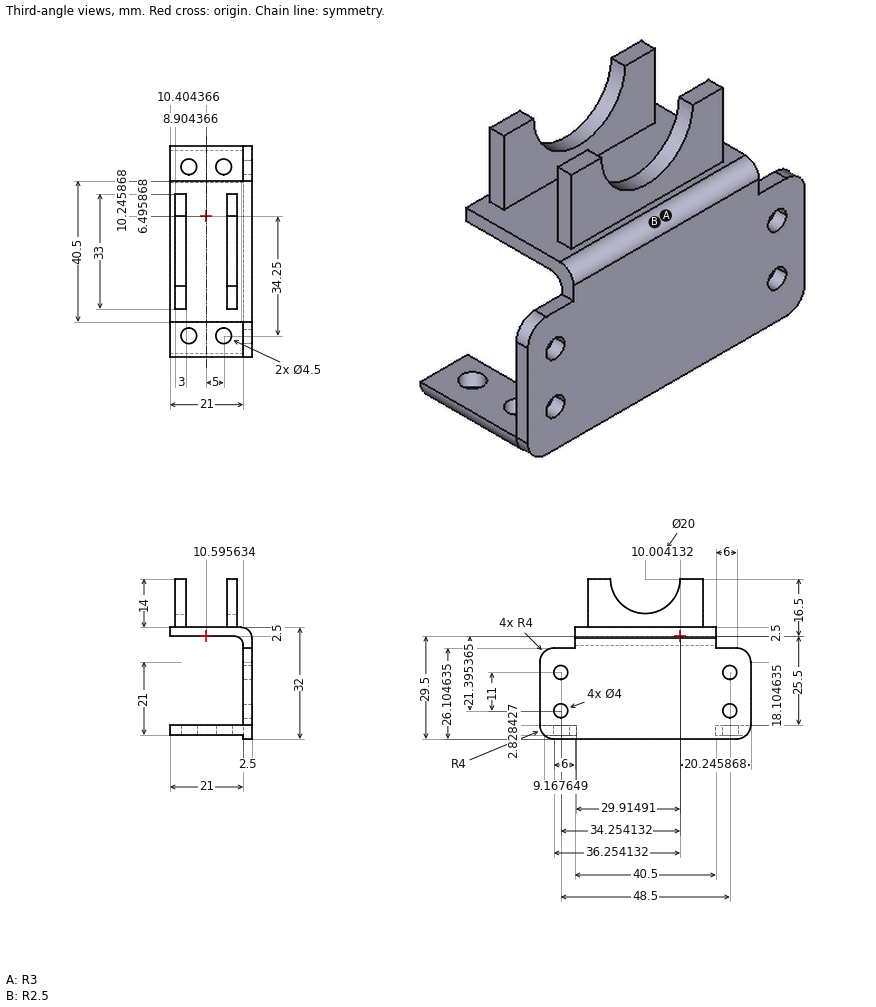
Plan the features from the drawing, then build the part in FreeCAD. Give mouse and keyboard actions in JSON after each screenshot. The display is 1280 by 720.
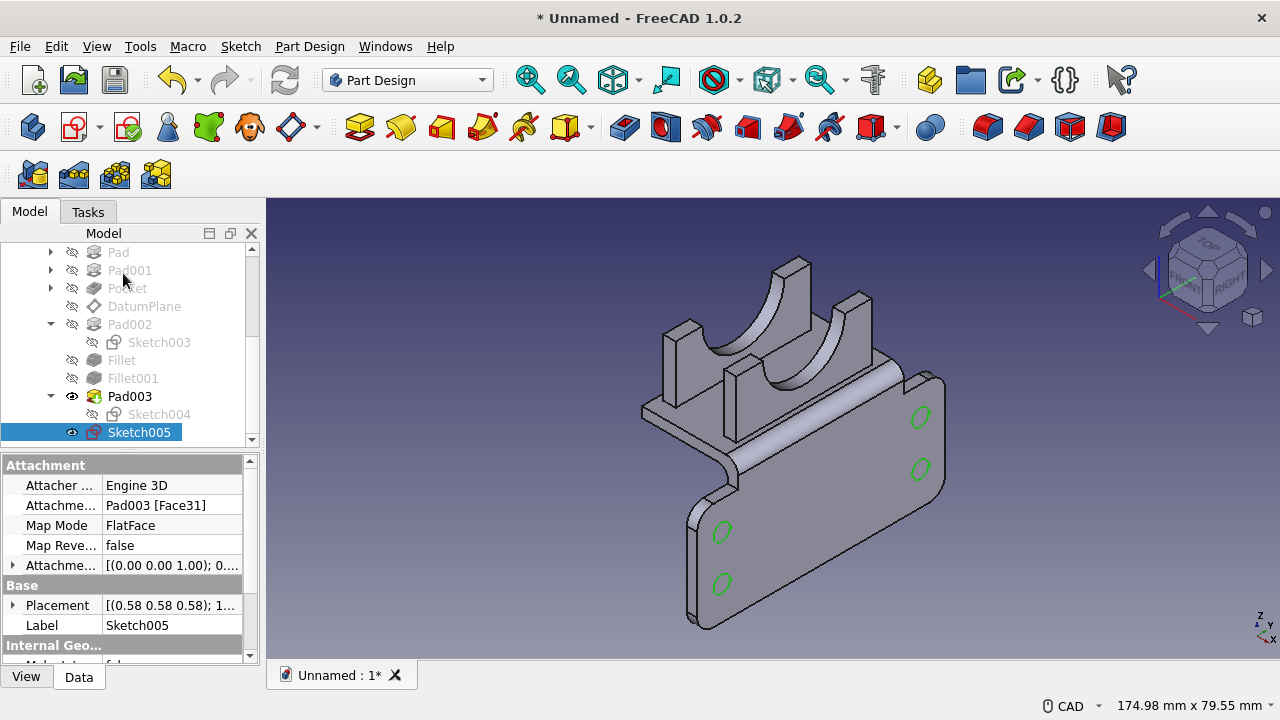
{"action": "left_click", "coordinate": [625, 128]}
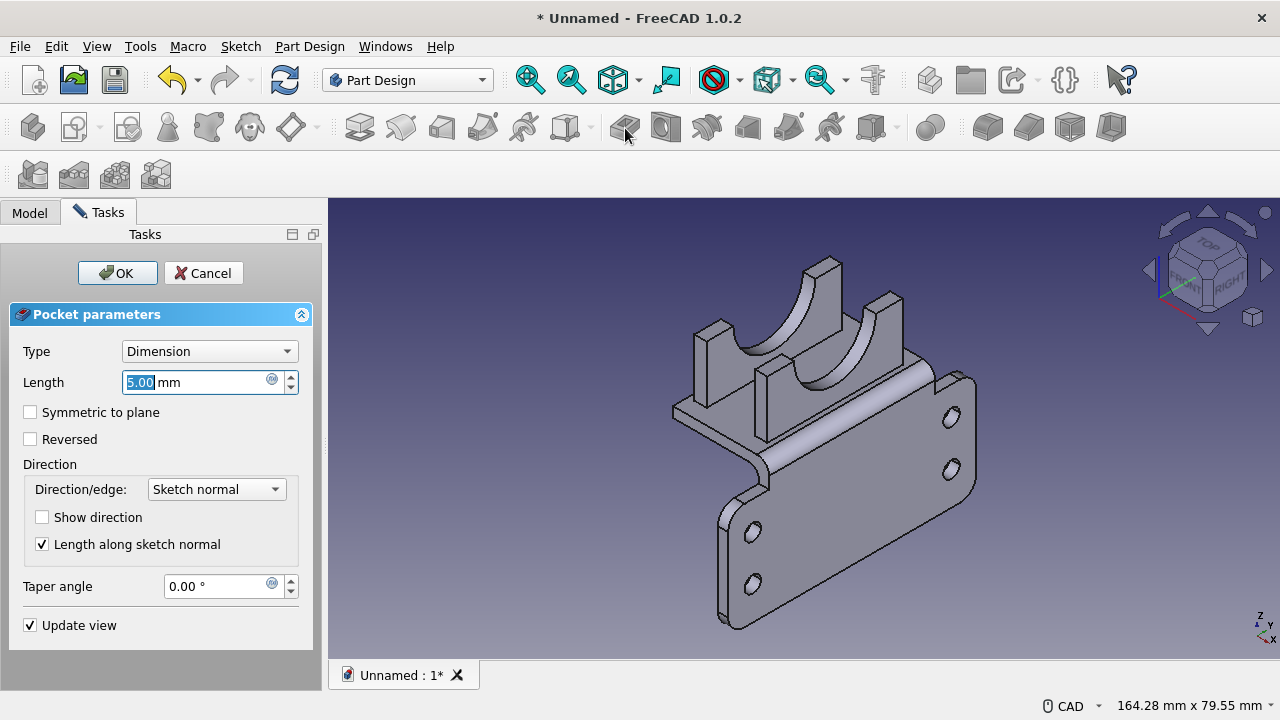
{"action": "left_click", "coordinate": [210, 352]}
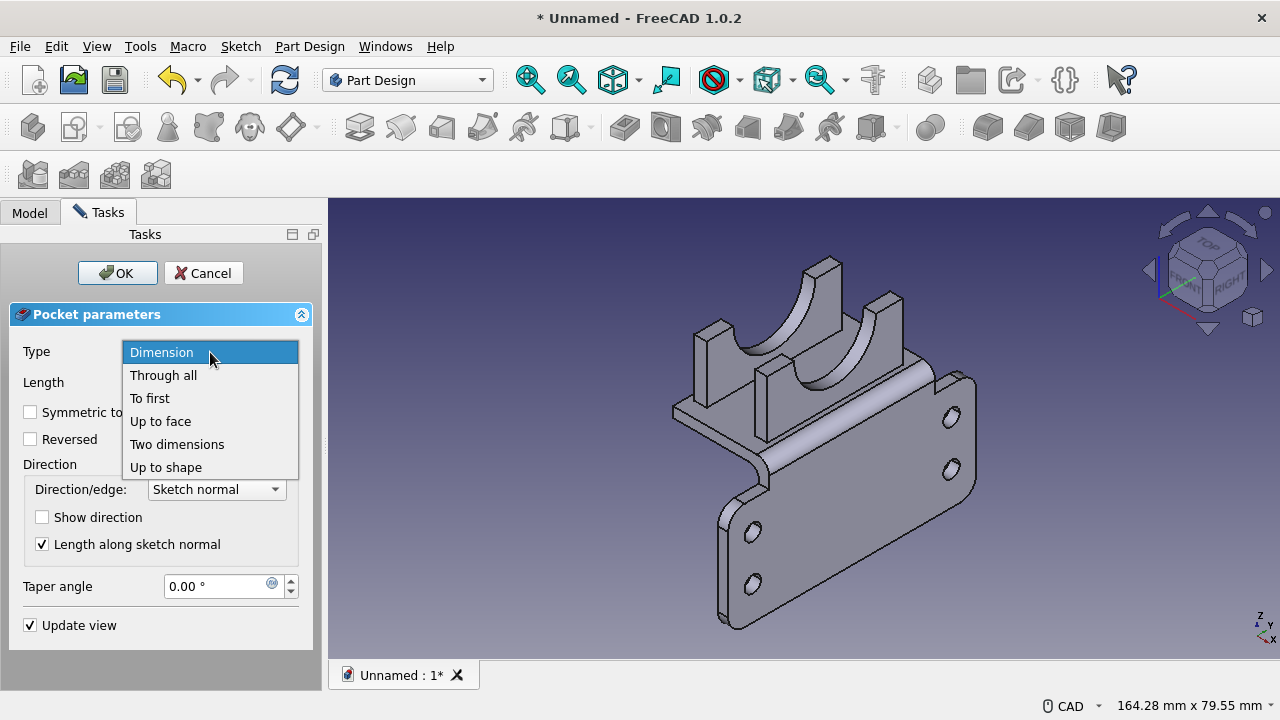
{"action": "left_click", "coordinate": [208, 376]}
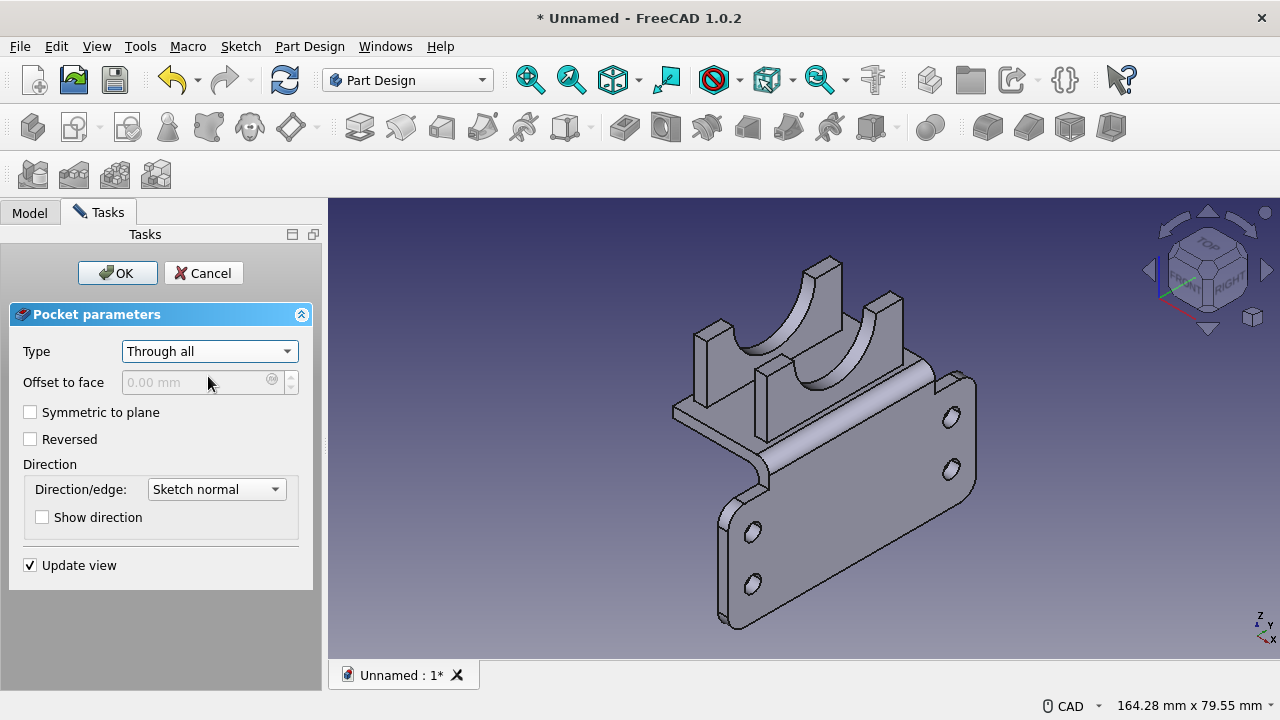
{"action": "left_click", "coordinate": [118, 273]}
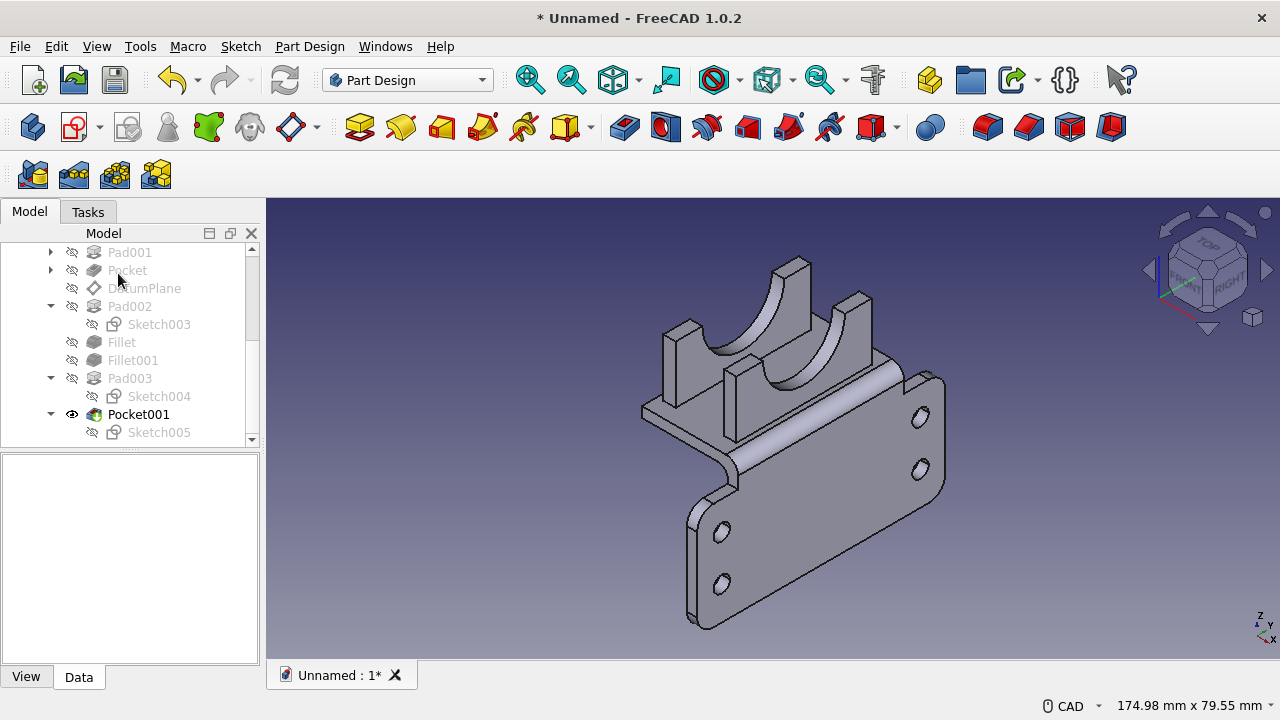
{"action": "key", "text": "6"}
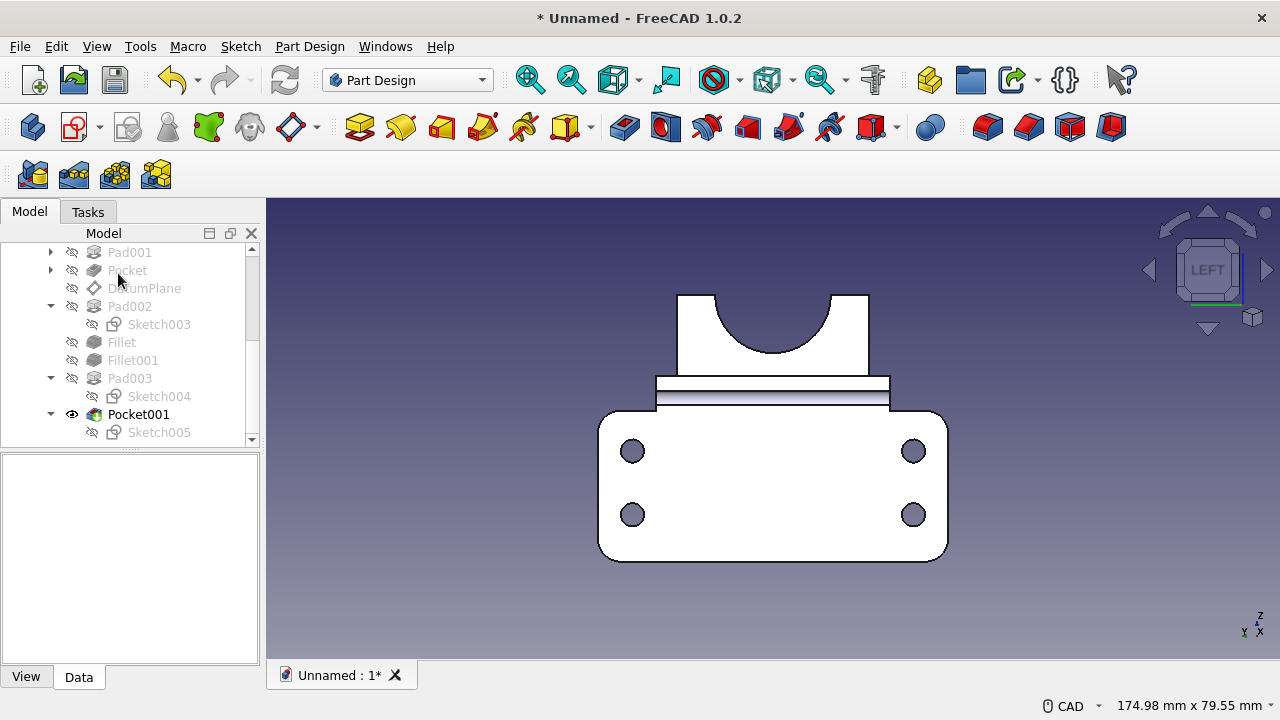
{"action": "left_click", "coordinate": [723, 483]}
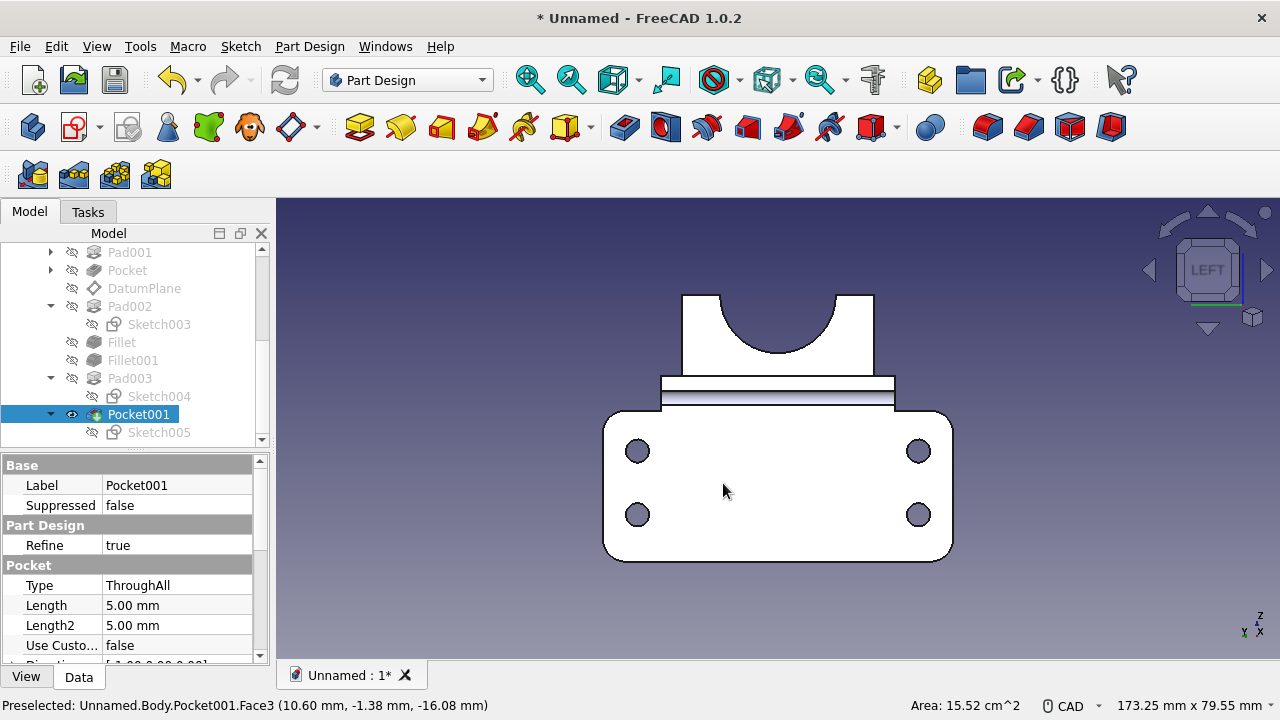
{"action": "left_click", "coordinate": [74, 128]}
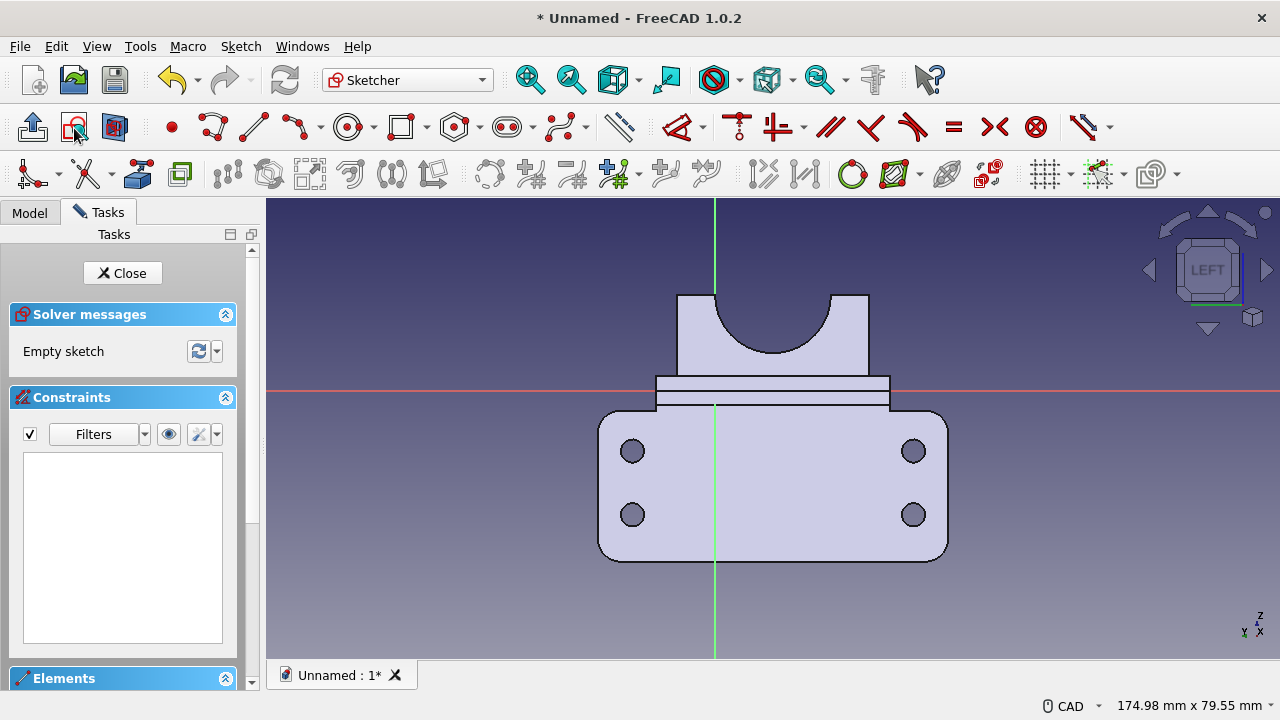
{"action": "left_click", "coordinate": [115, 128]}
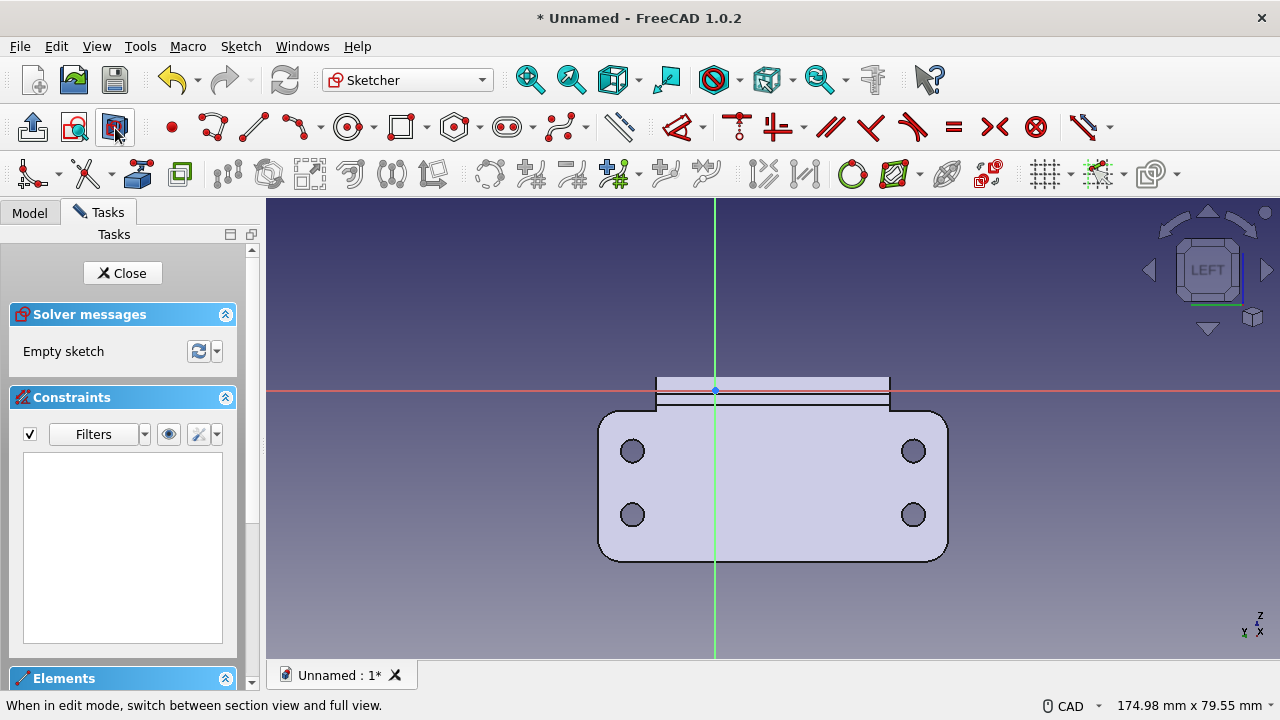
{"action": "scroll", "coordinate": [945, 562], "scroll_direction": "up", "scroll_amount": 11}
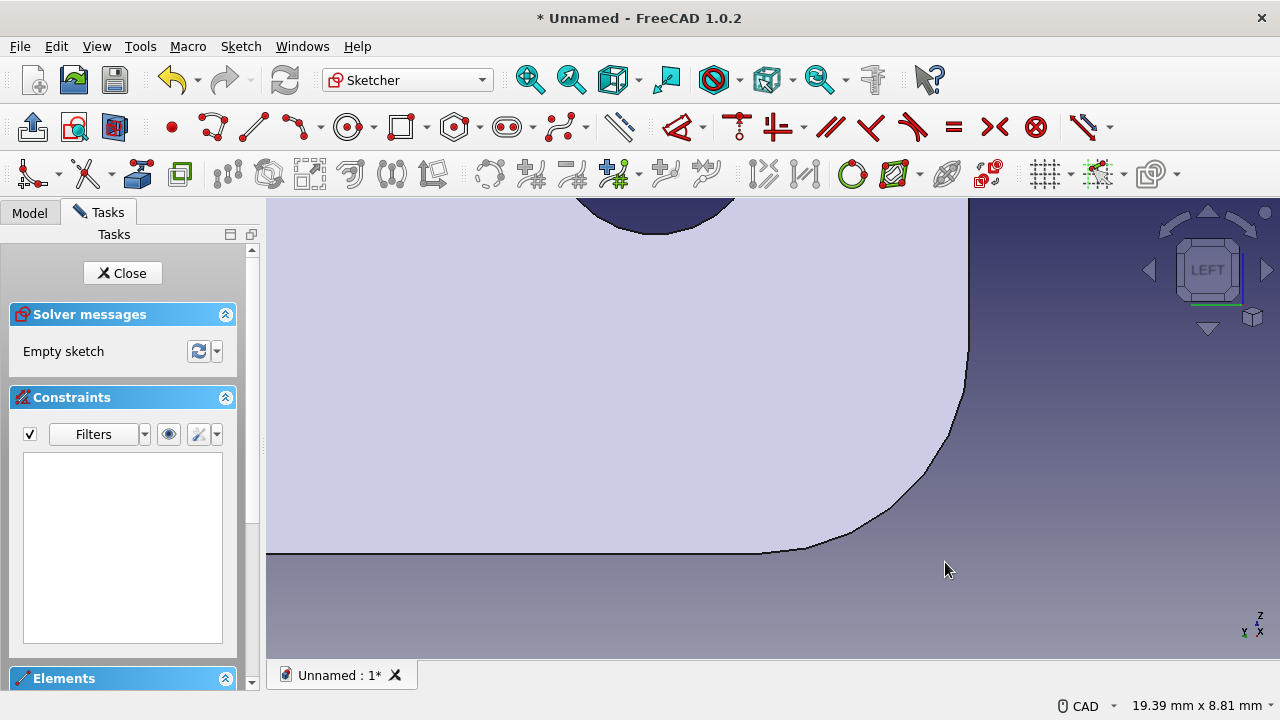
{"action": "left_click", "coordinate": [213, 128]}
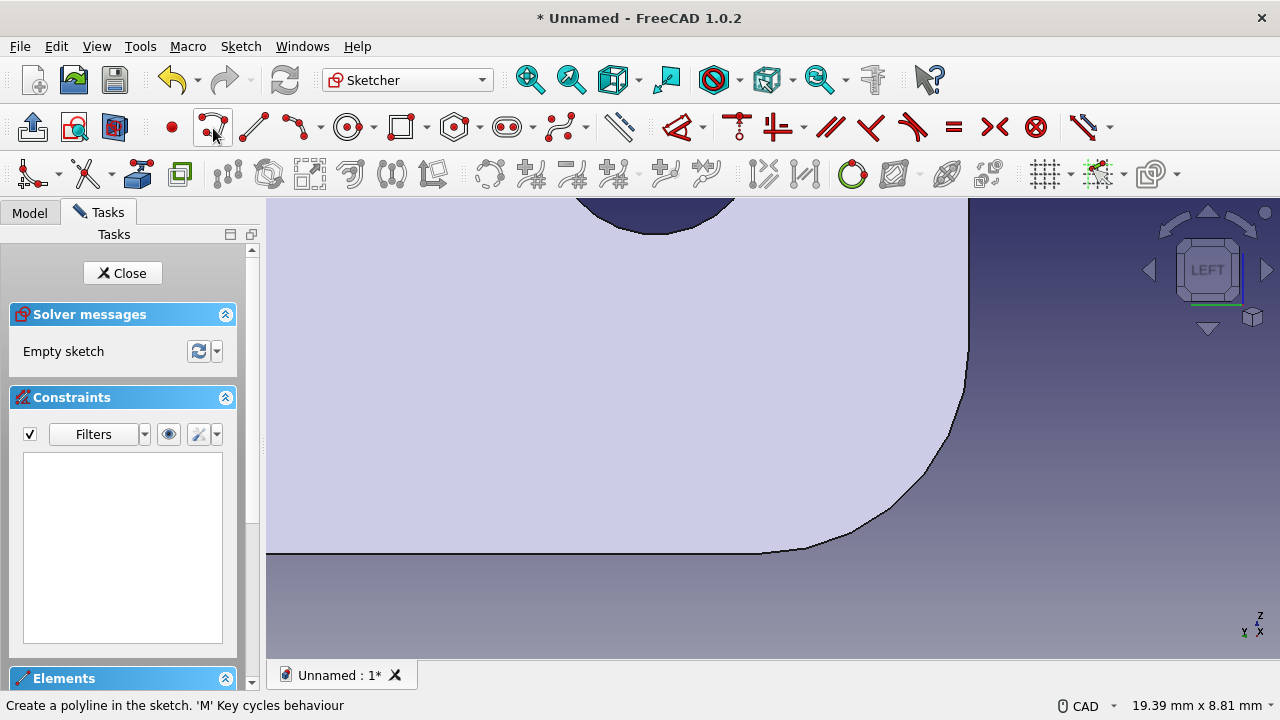
{"action": "left_click", "coordinate": [969, 345]}
{"action": "left_click", "coordinate": [429, 345]}
{"action": "left_click", "coordinate": [429, 492]}
{"action": "left_click", "coordinate": [908, 492]}
{"action": "right_click", "coordinate": [908, 492]}